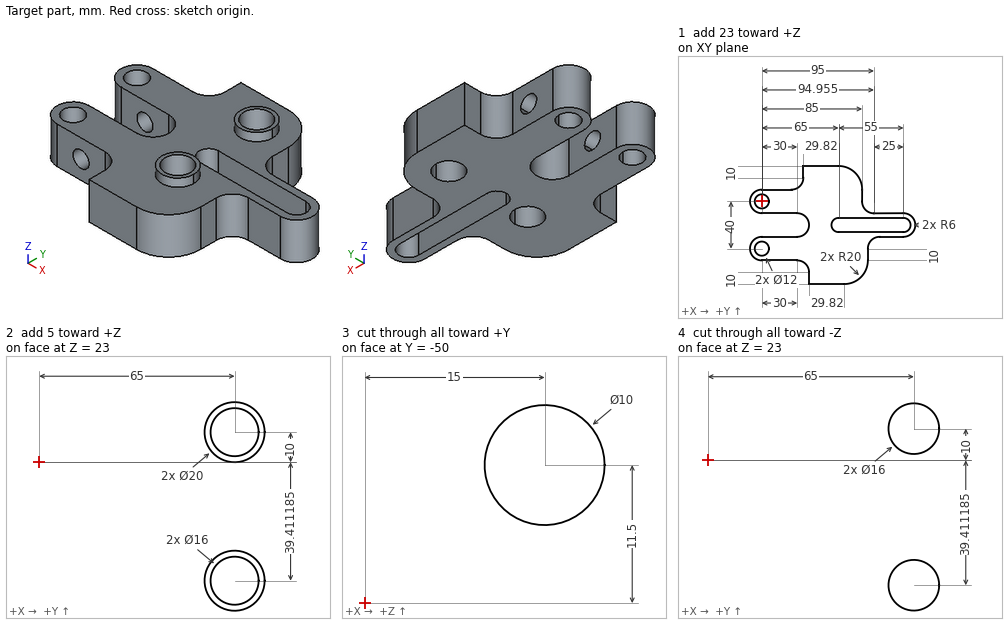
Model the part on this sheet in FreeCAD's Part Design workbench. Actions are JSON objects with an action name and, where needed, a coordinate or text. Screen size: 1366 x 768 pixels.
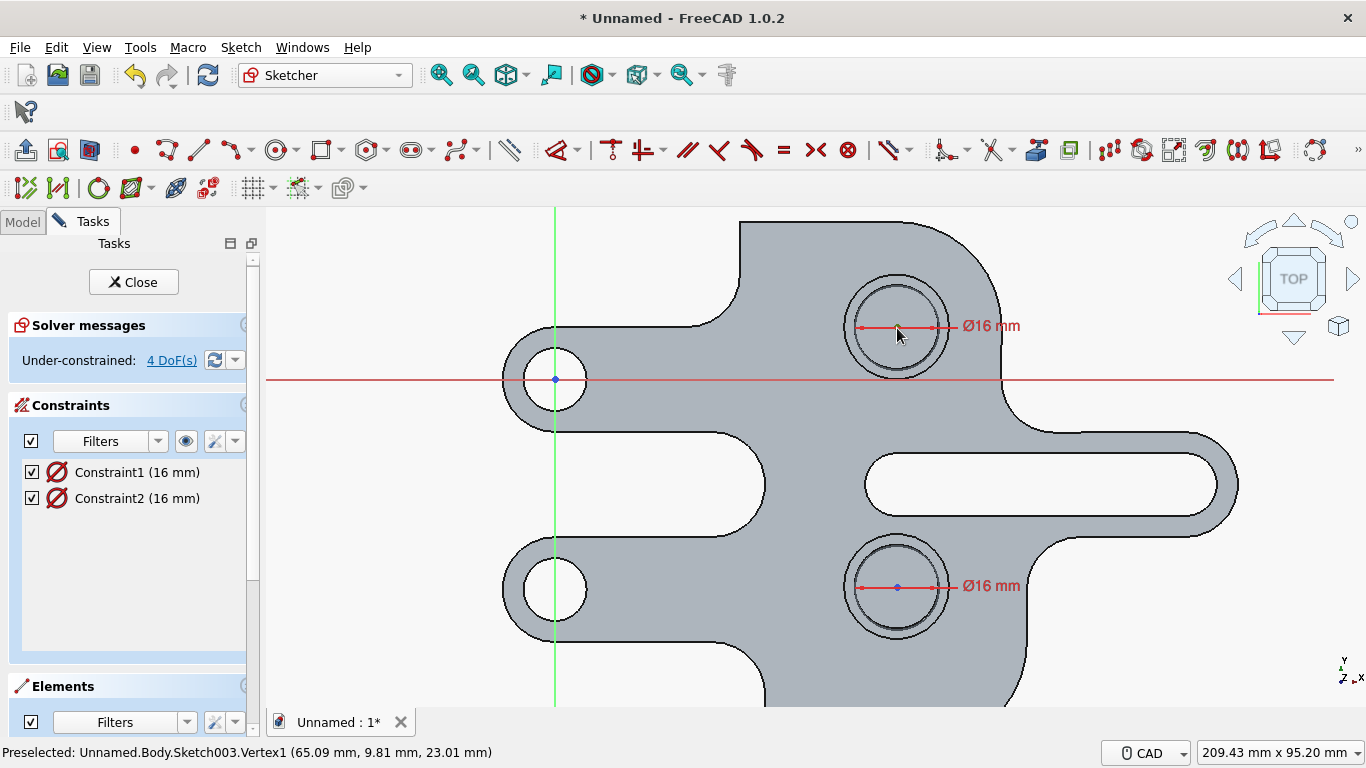
{"action": "left_click", "coordinate": [897, 588]}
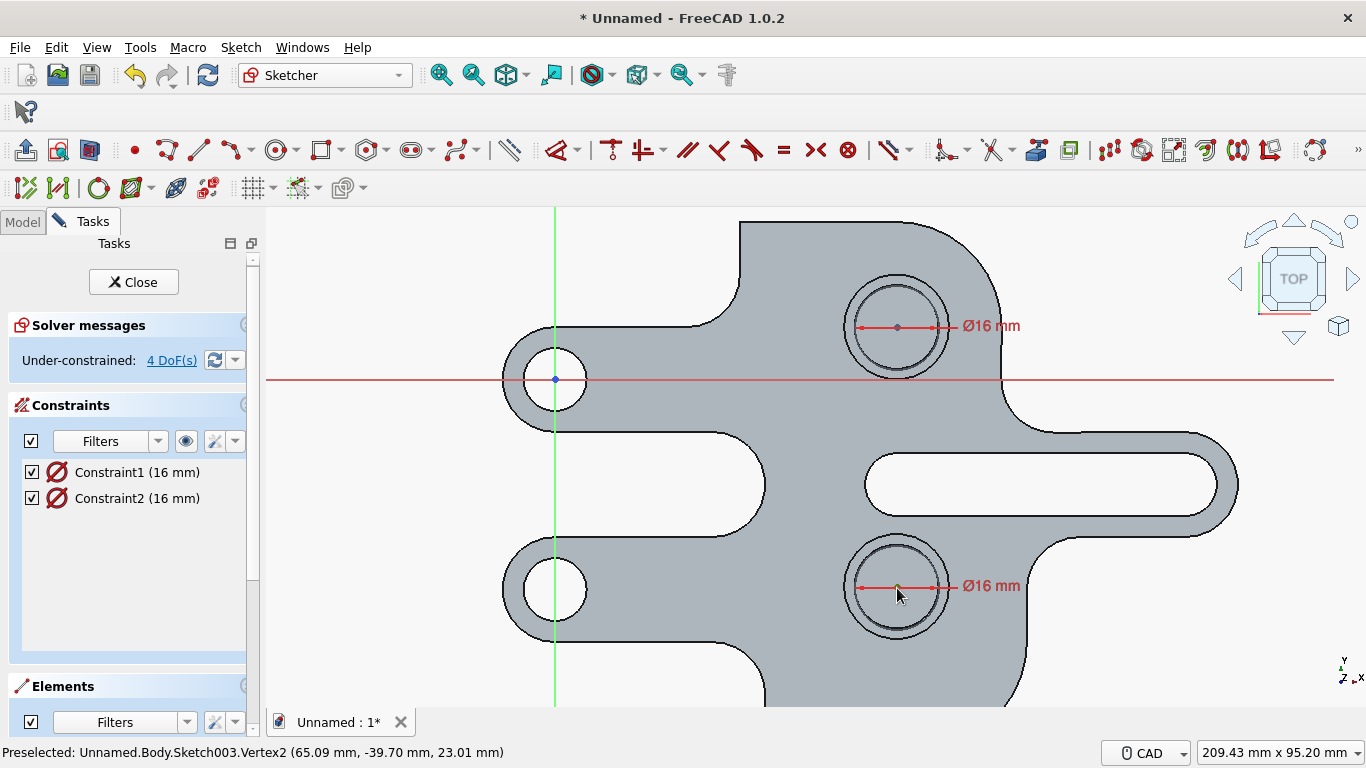
{"action": "left_click", "coordinate": [666, 150]}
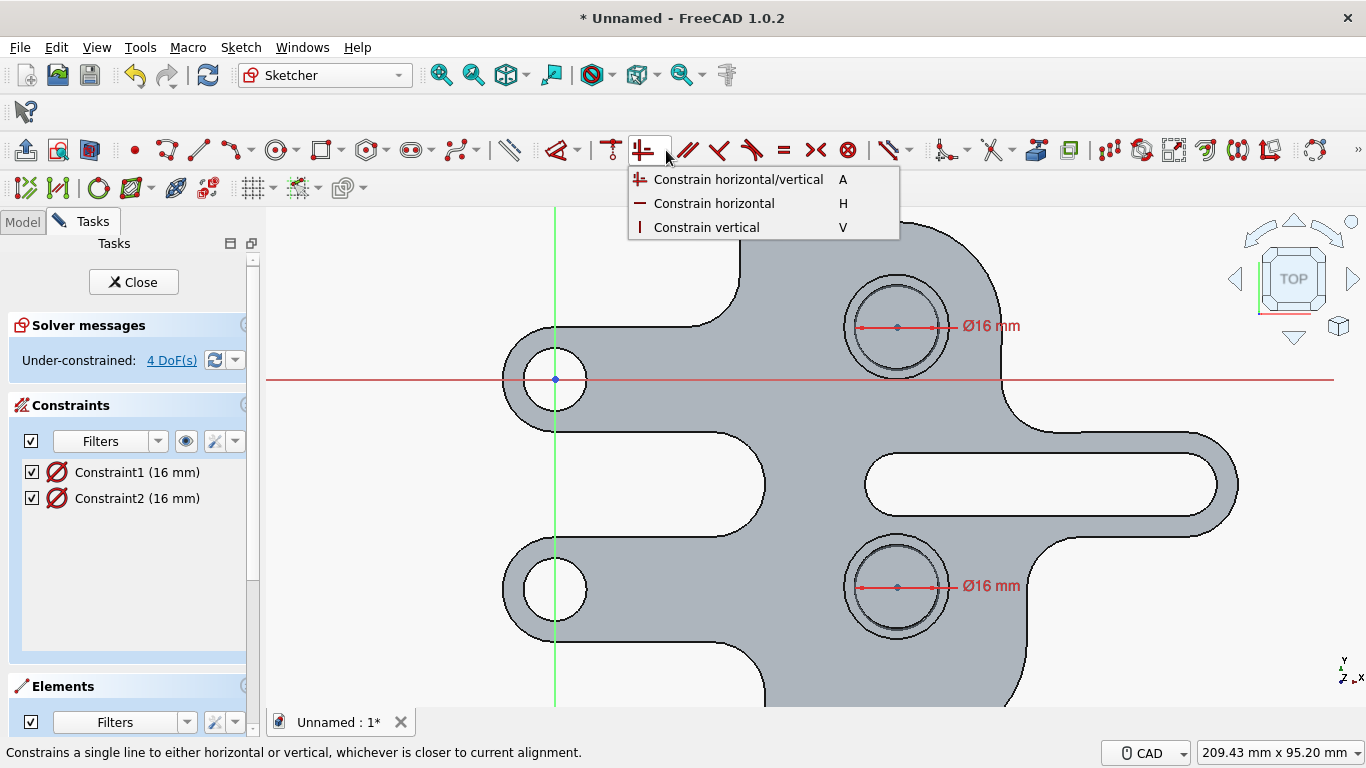
{"action": "left_click", "coordinate": [764, 227]}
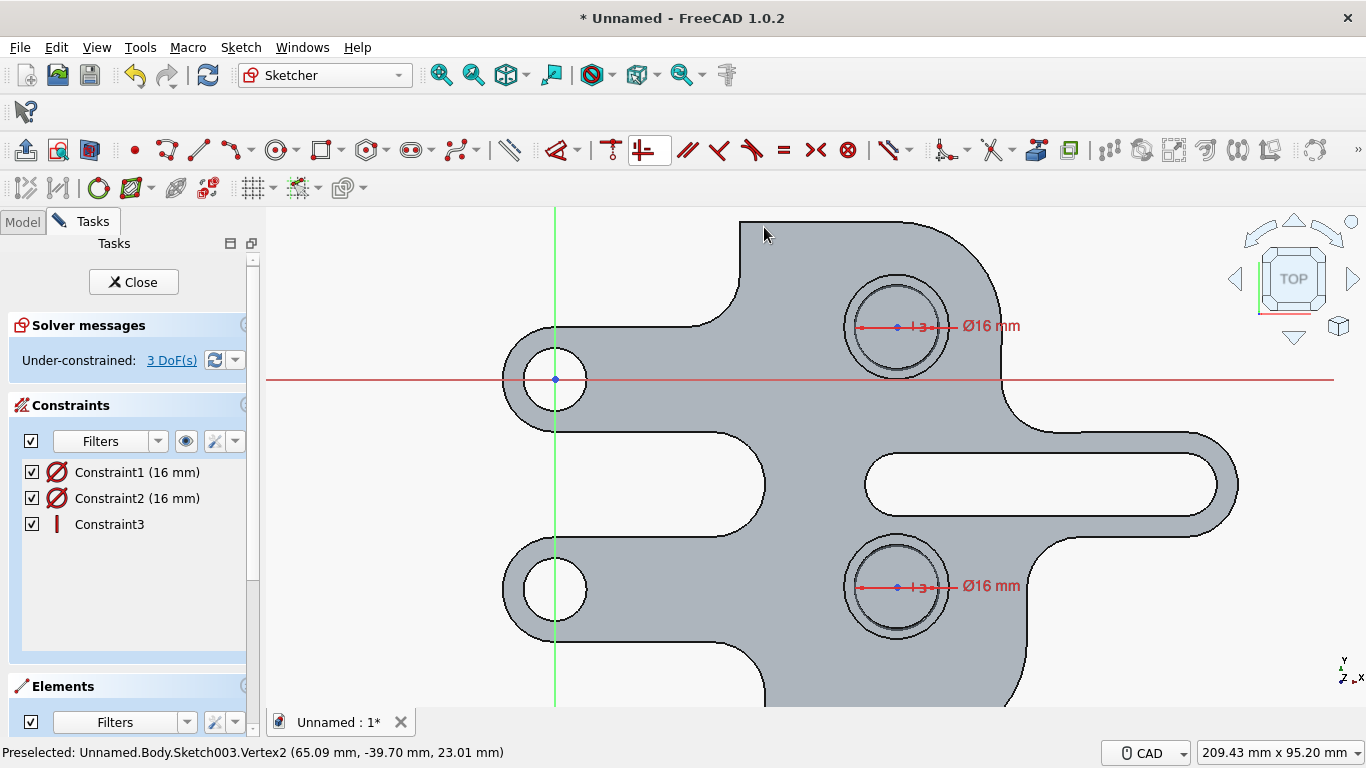
{"action": "left_click", "coordinate": [556, 150]}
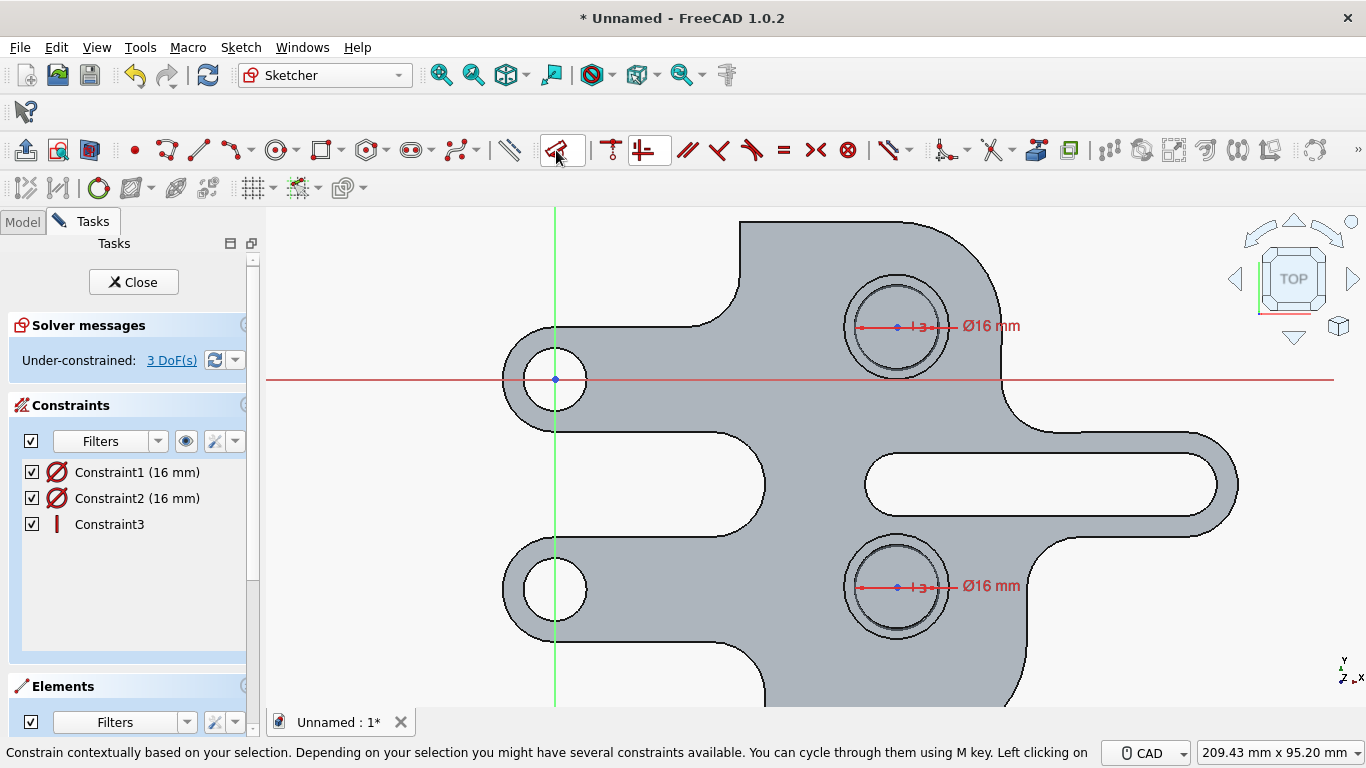
{"action": "left_click", "coordinate": [897, 328]}
{"action": "left_click", "coordinate": [726, 294]}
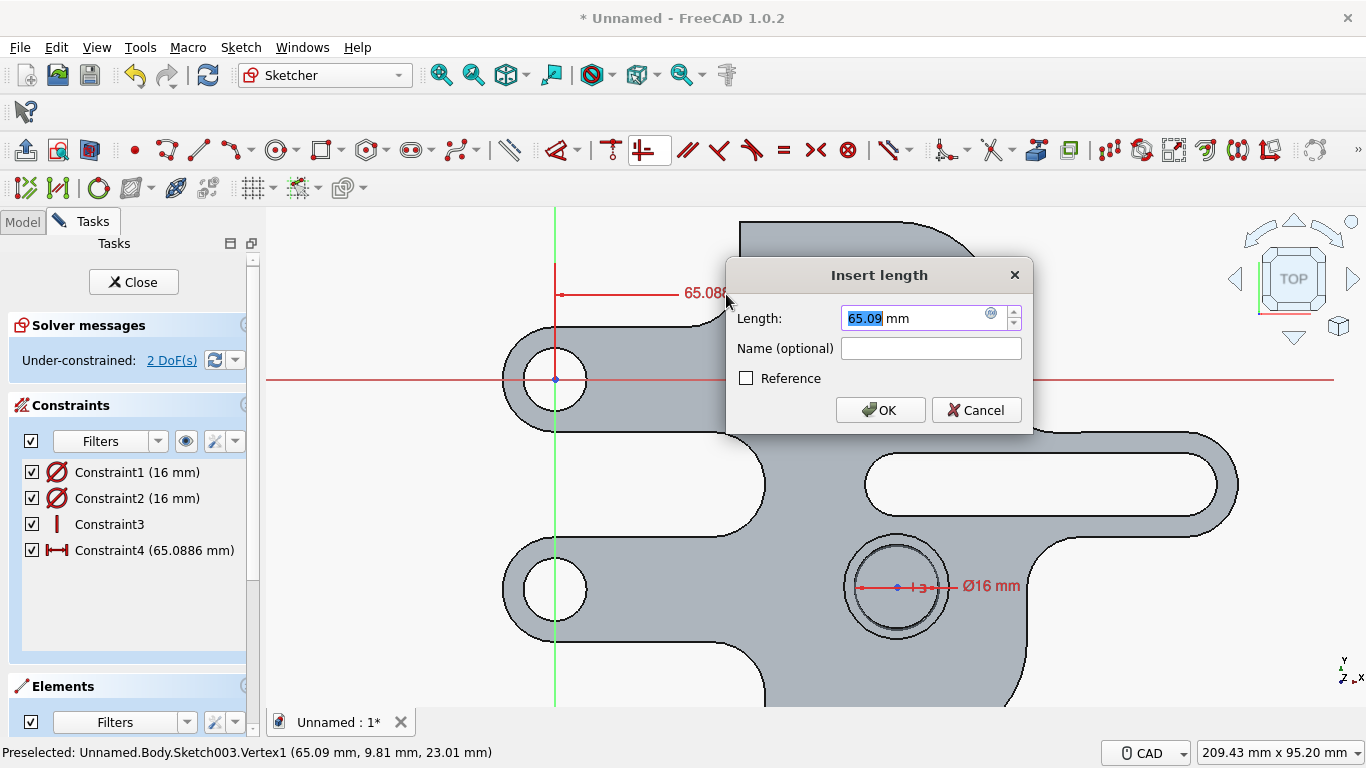
{"action": "type", "text": "65"}
{"action": "key", "text": "Return"}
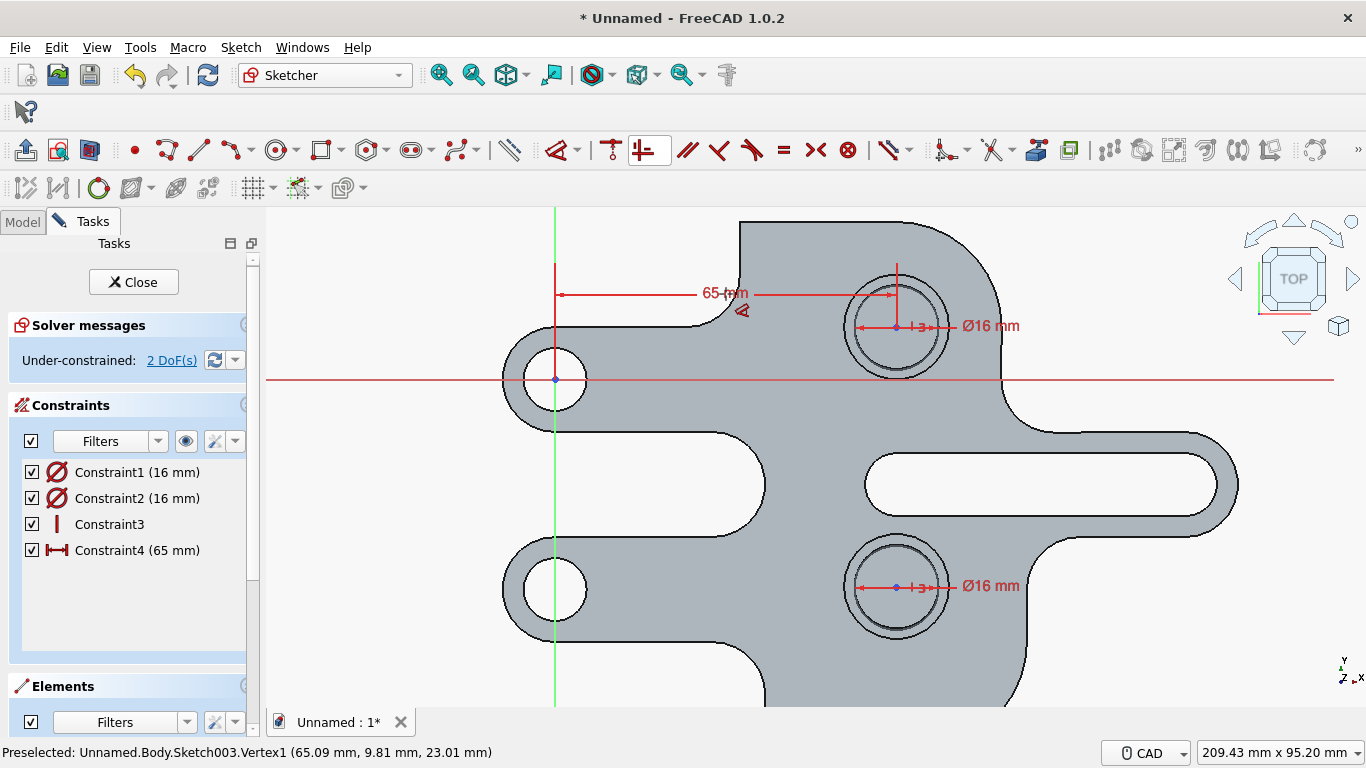
{"action": "left_click", "coordinate": [897, 328]}
{"action": "left_click", "coordinate": [521, 354]}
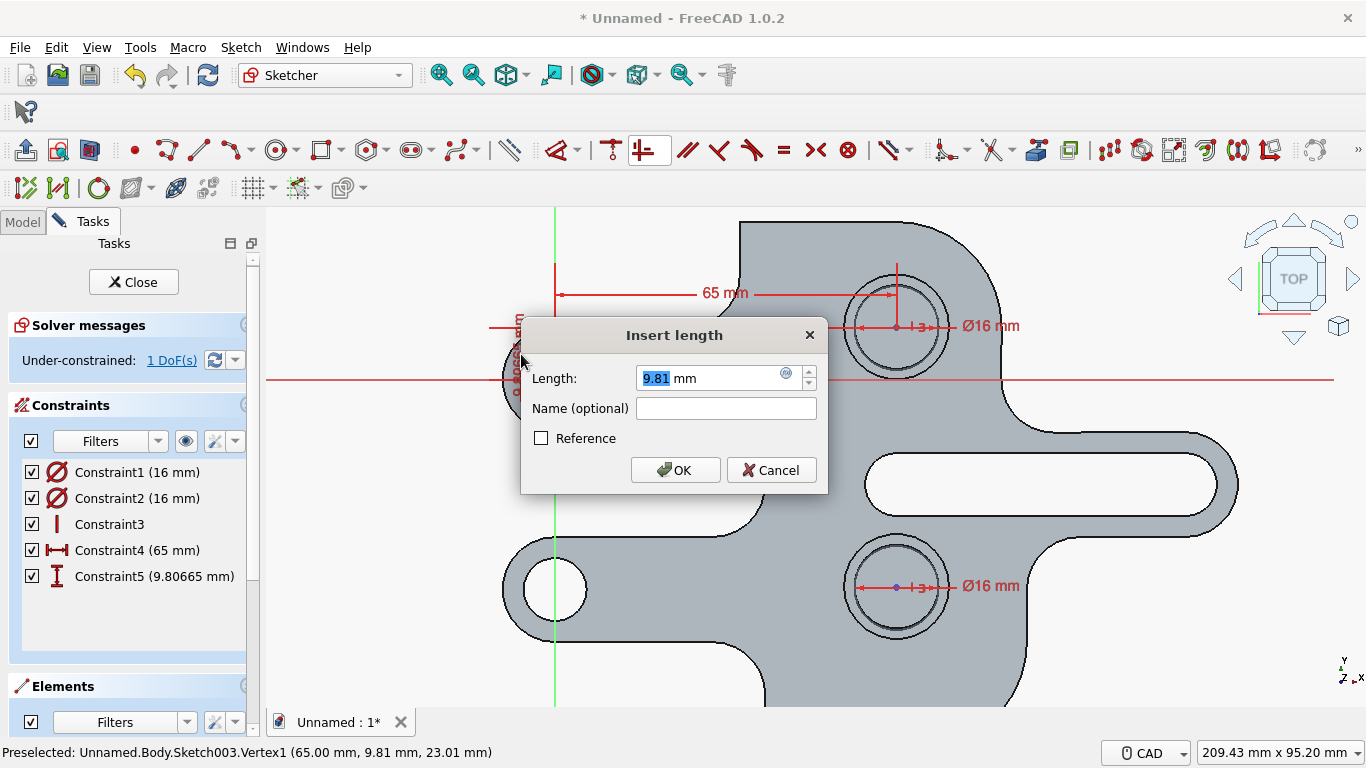
{"action": "type", "text": "10"}
{"action": "key", "text": "Return"}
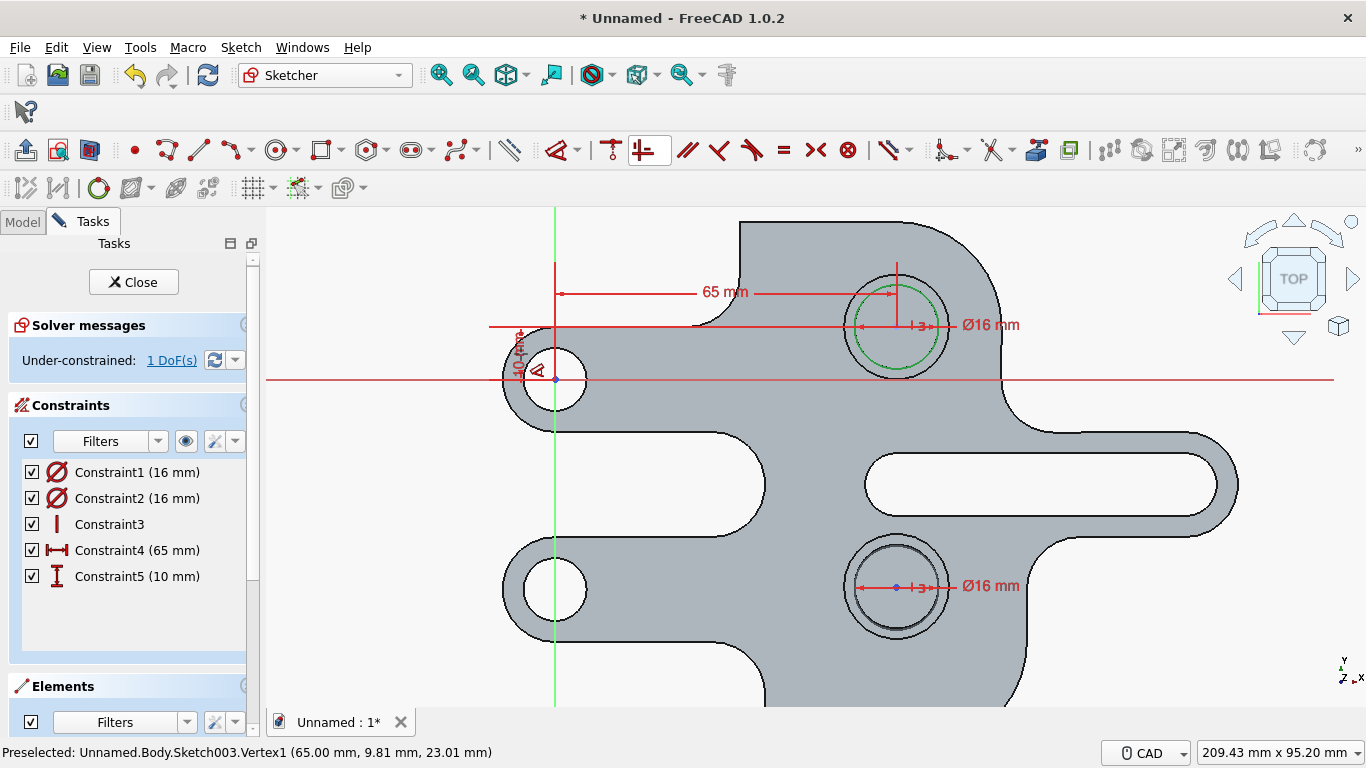
{"action": "left_click", "coordinate": [897, 588]}
{"action": "left_click", "coordinate": [521, 484]}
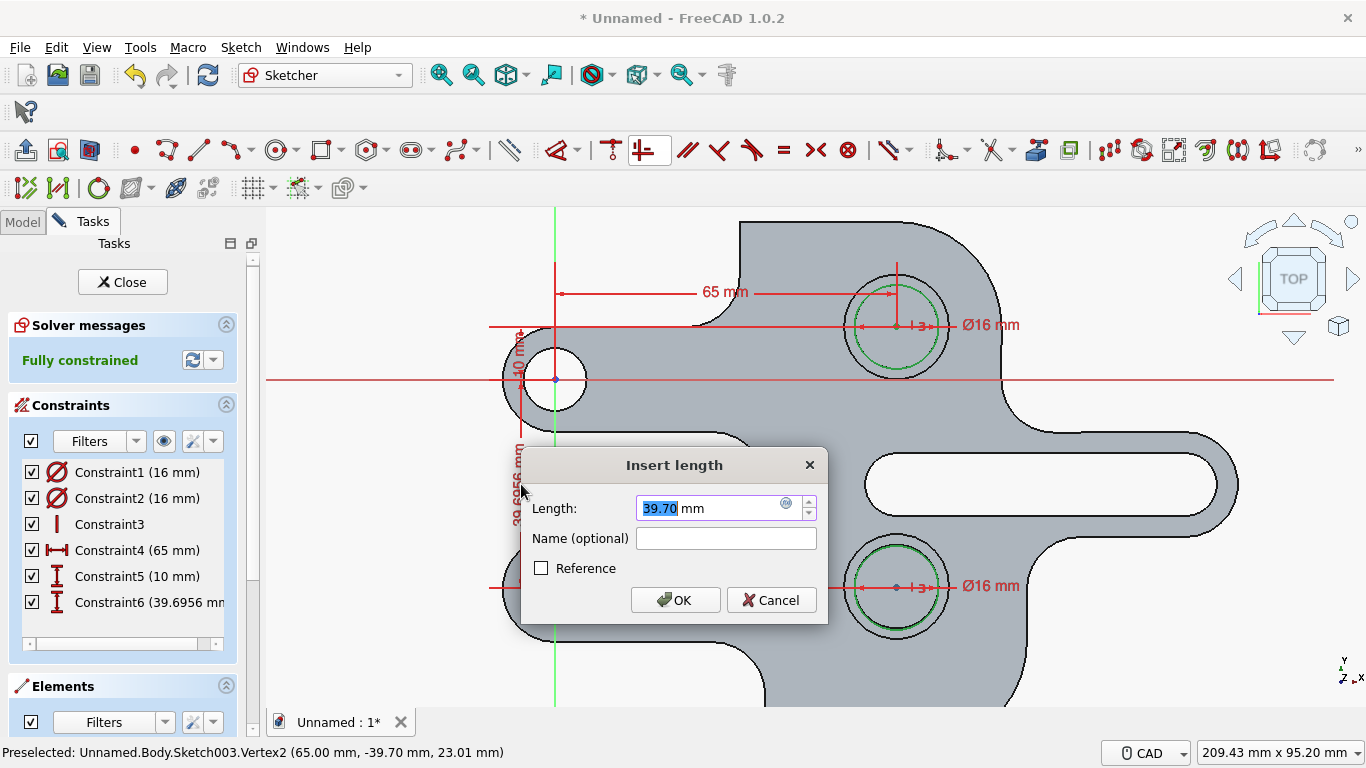
{"action": "type", "text": "39.411185"}
{"action": "key", "text": "Return"}
{"action": "key", "text": "Escape"}